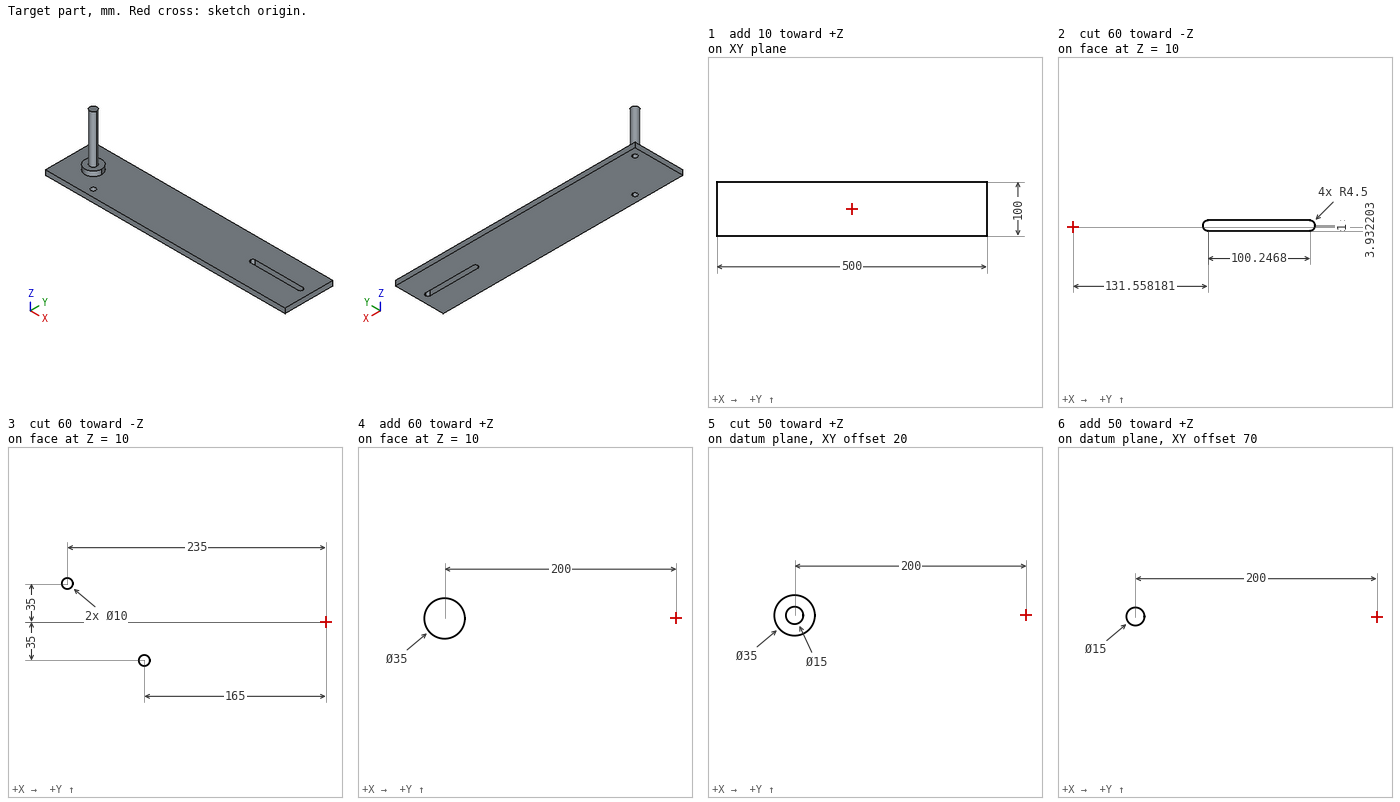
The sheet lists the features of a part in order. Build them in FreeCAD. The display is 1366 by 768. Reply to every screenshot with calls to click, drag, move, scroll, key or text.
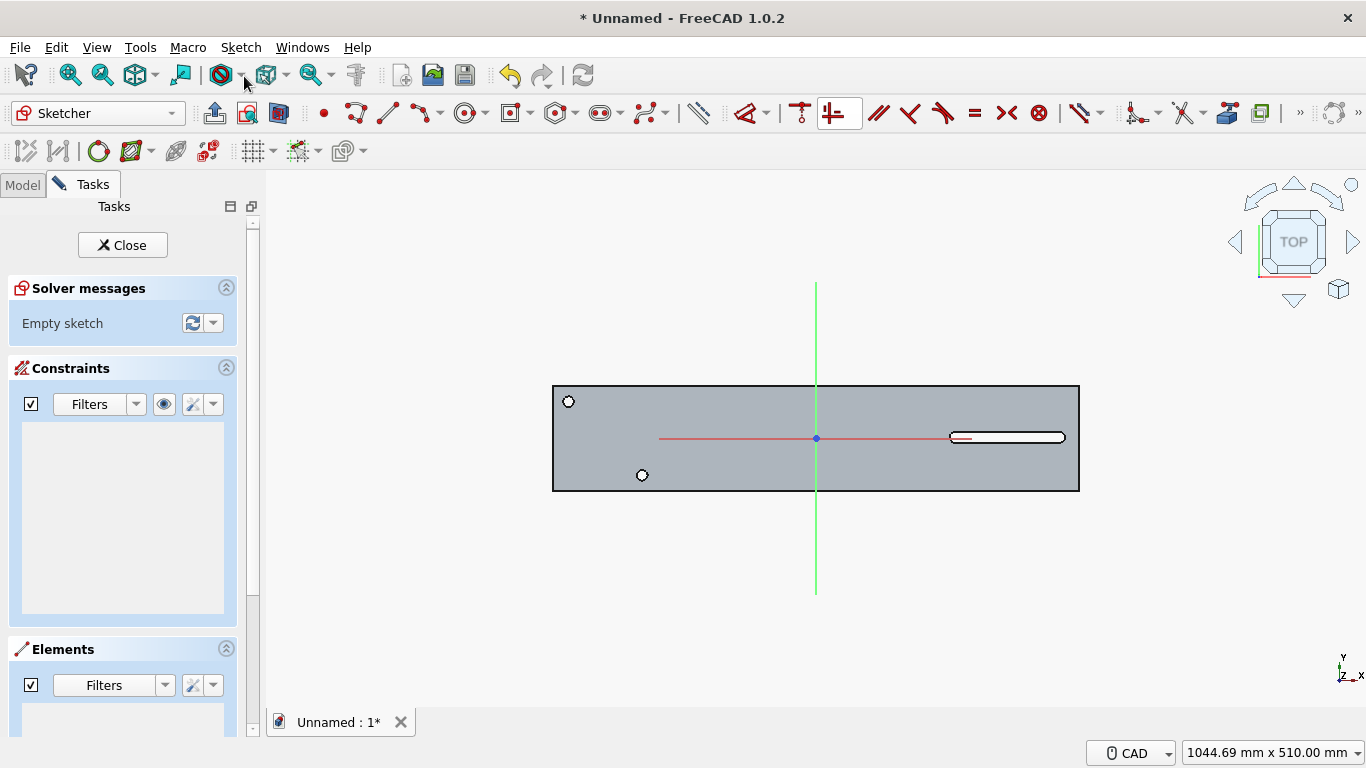
scroll(588, 438, up, 11)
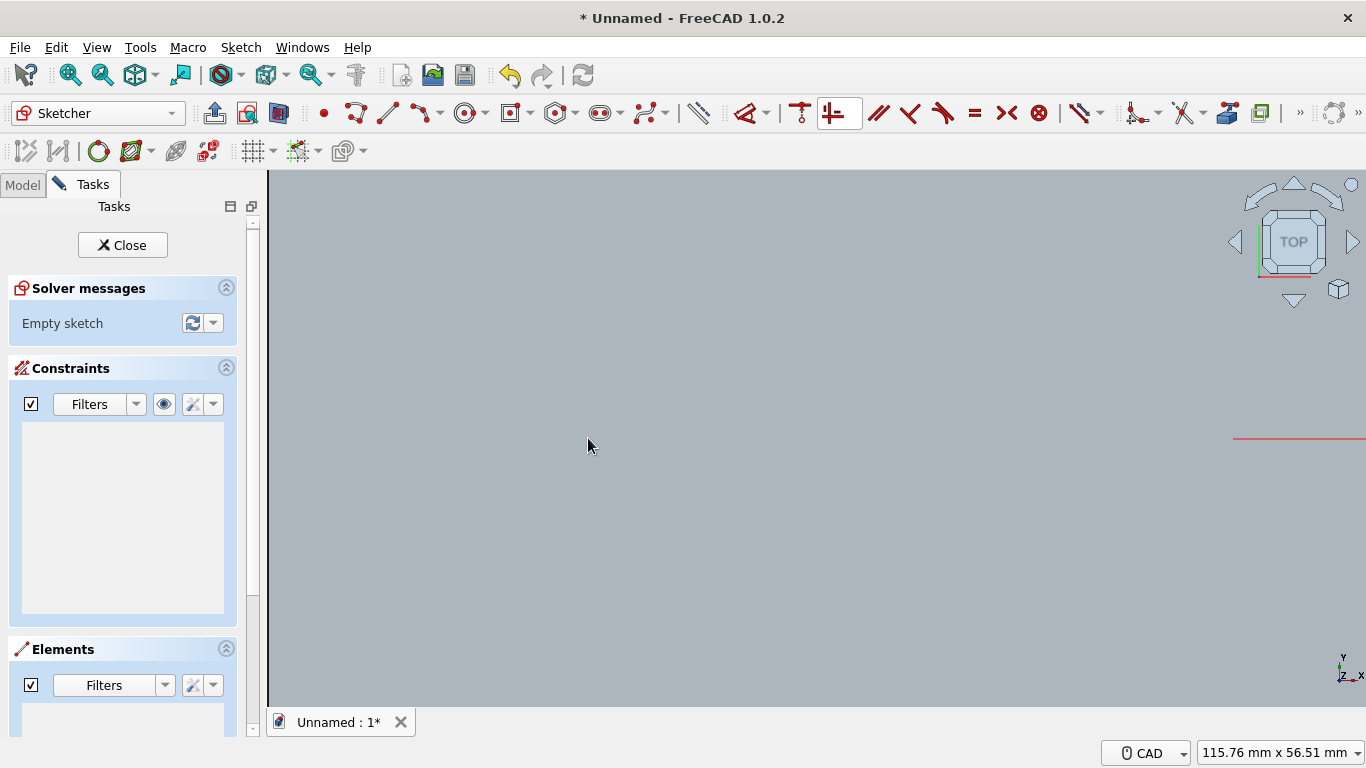
click(466, 114)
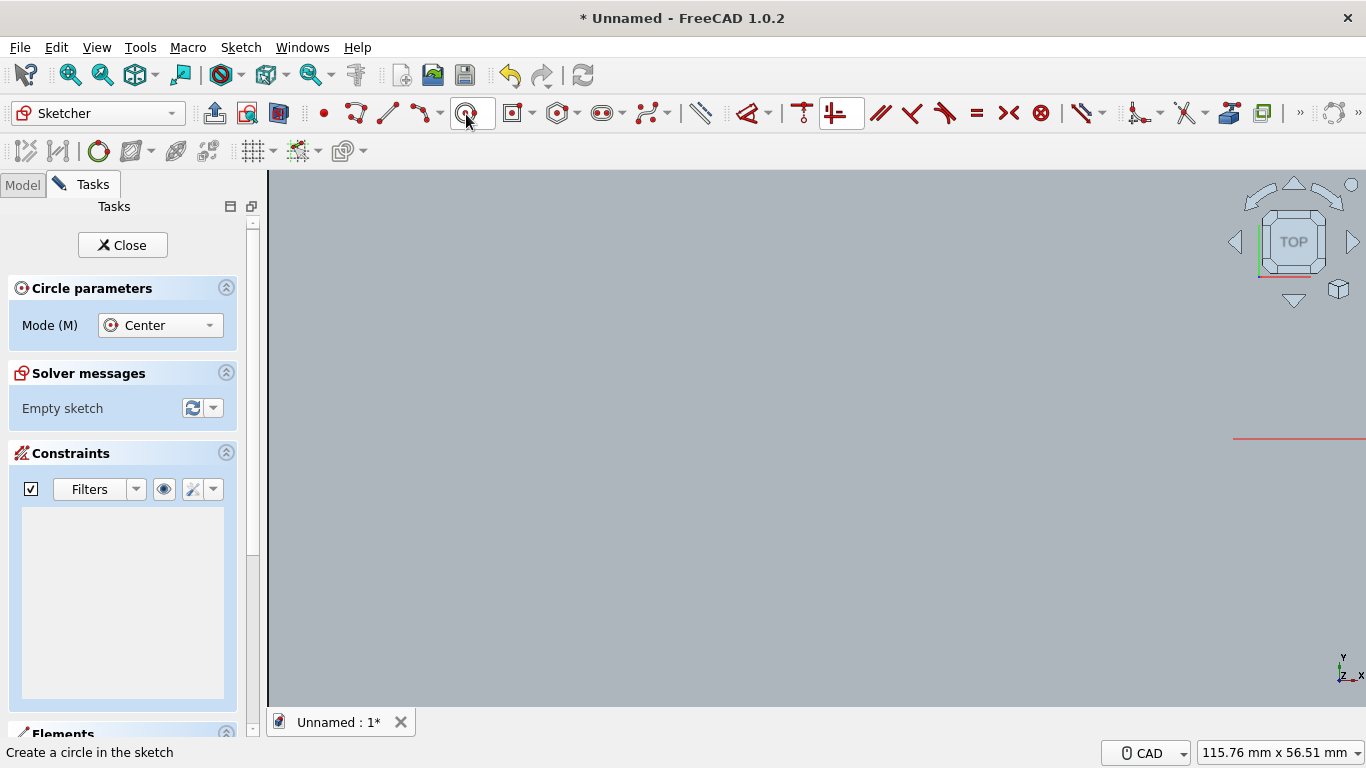
click(743, 438)
move(860, 321)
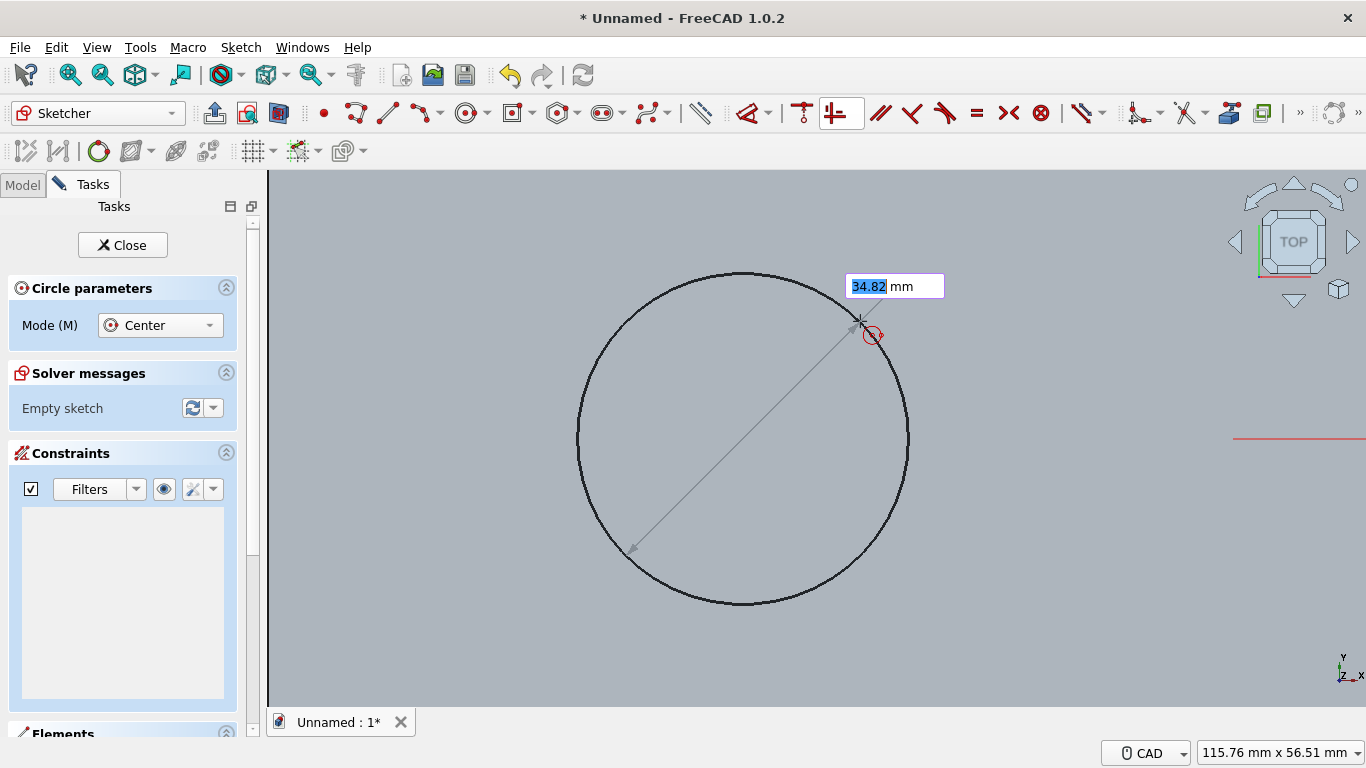
text(35)
key(Return)
key(Escape)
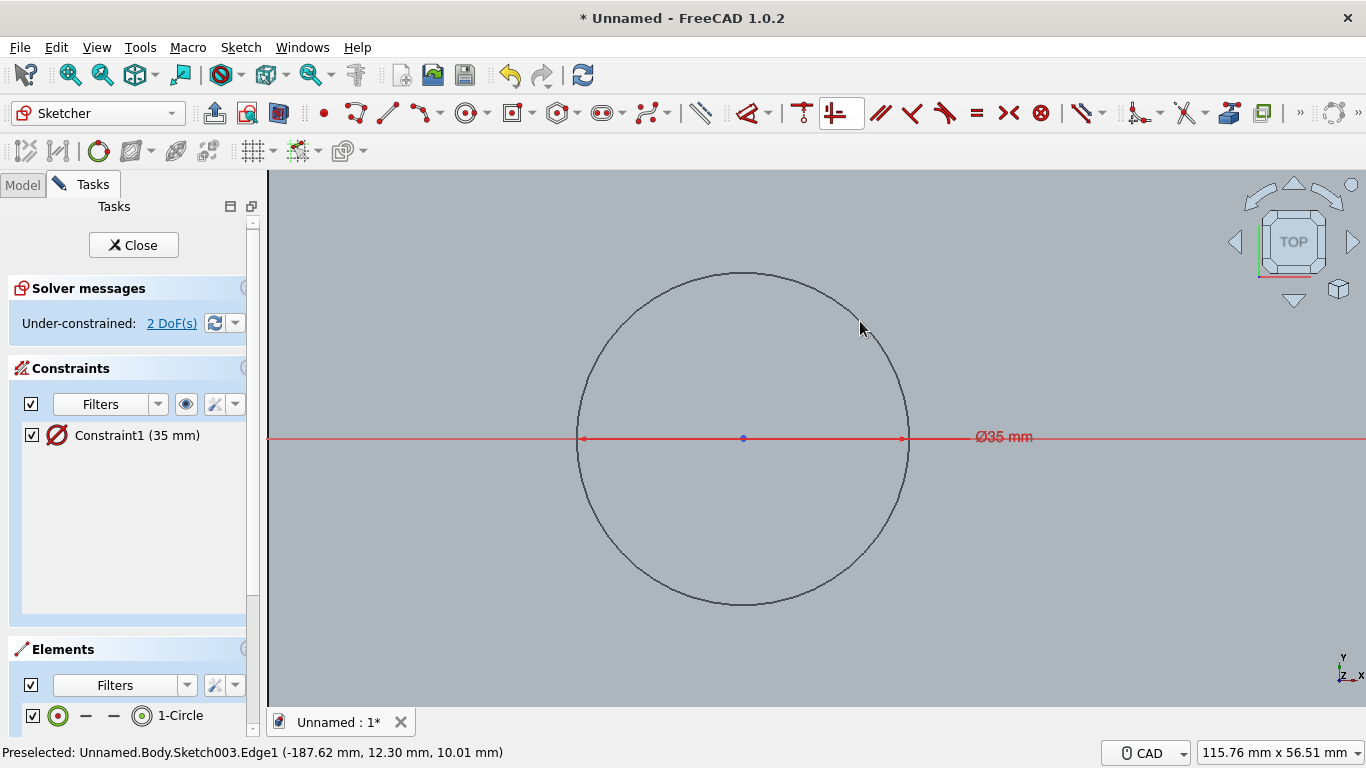
click(743, 439)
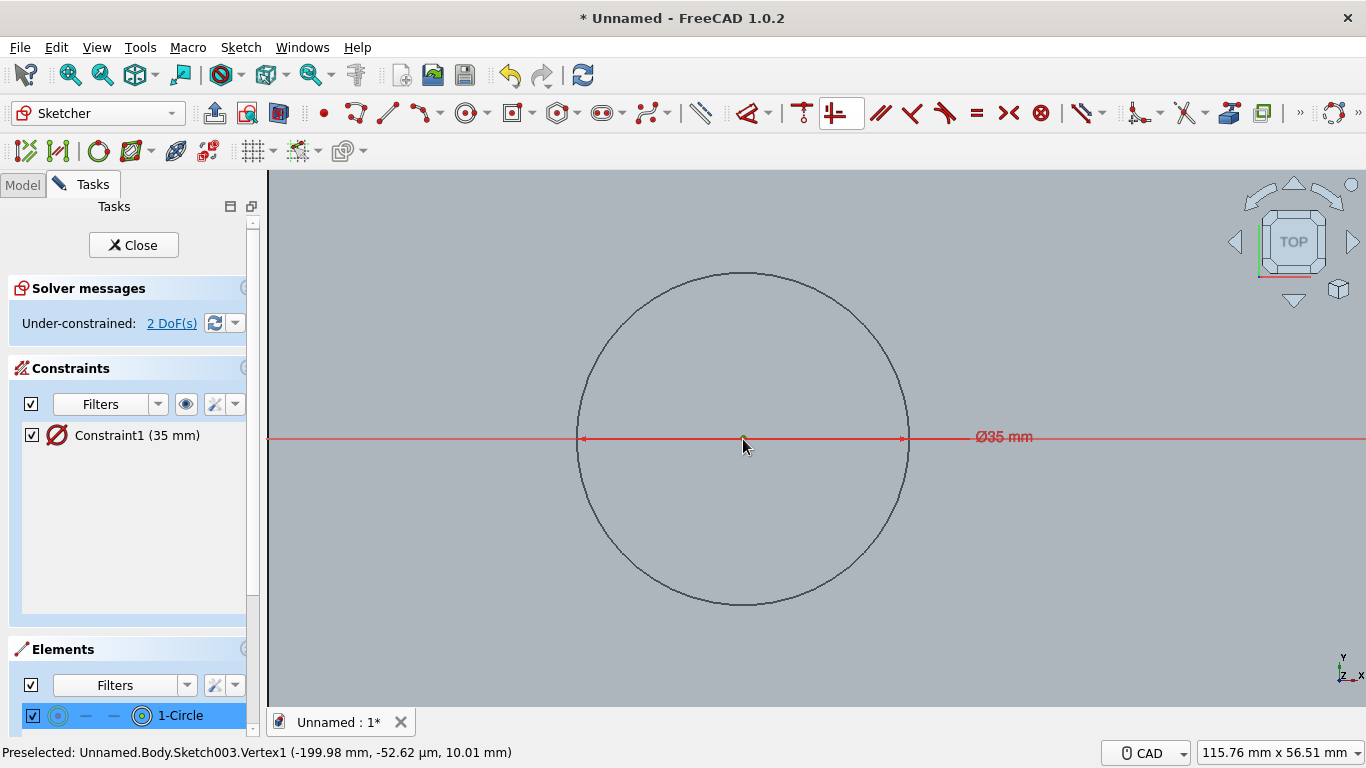
click(359, 438)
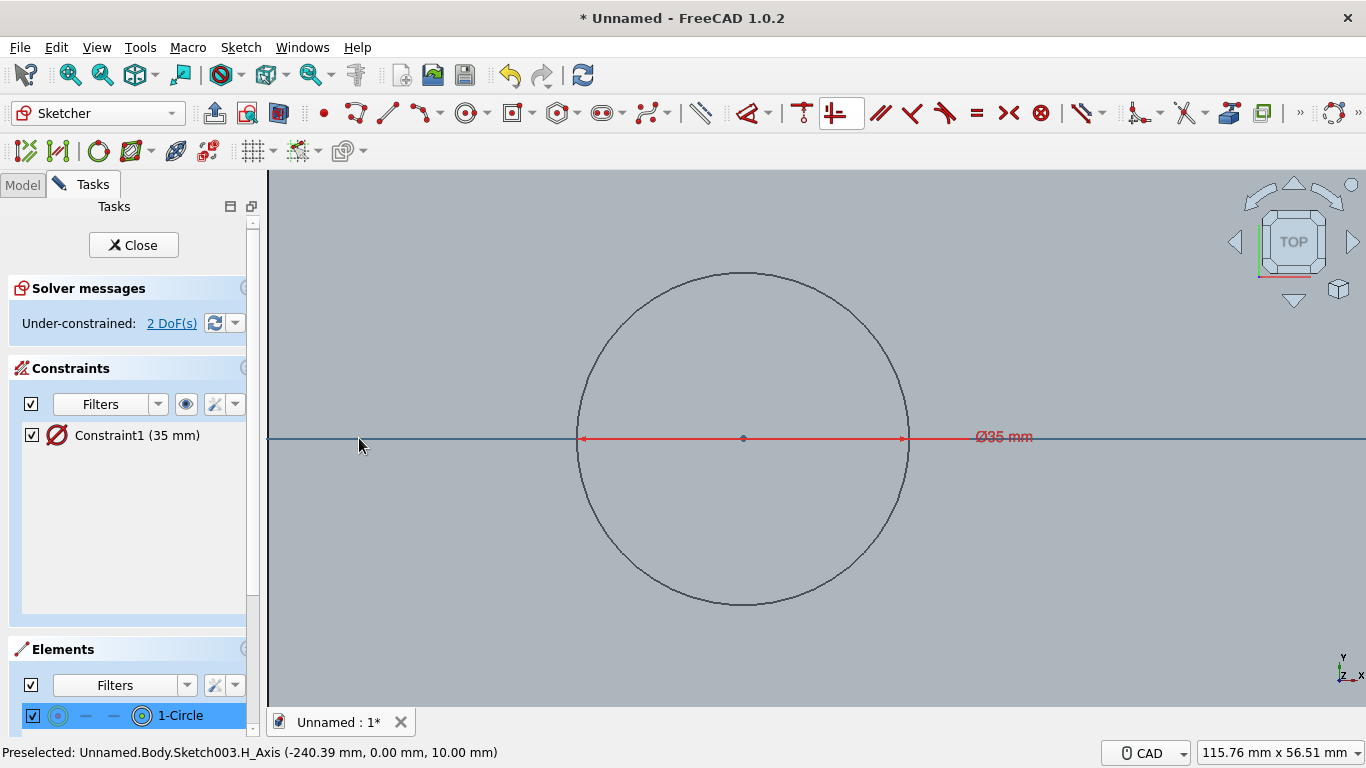
click(802, 114)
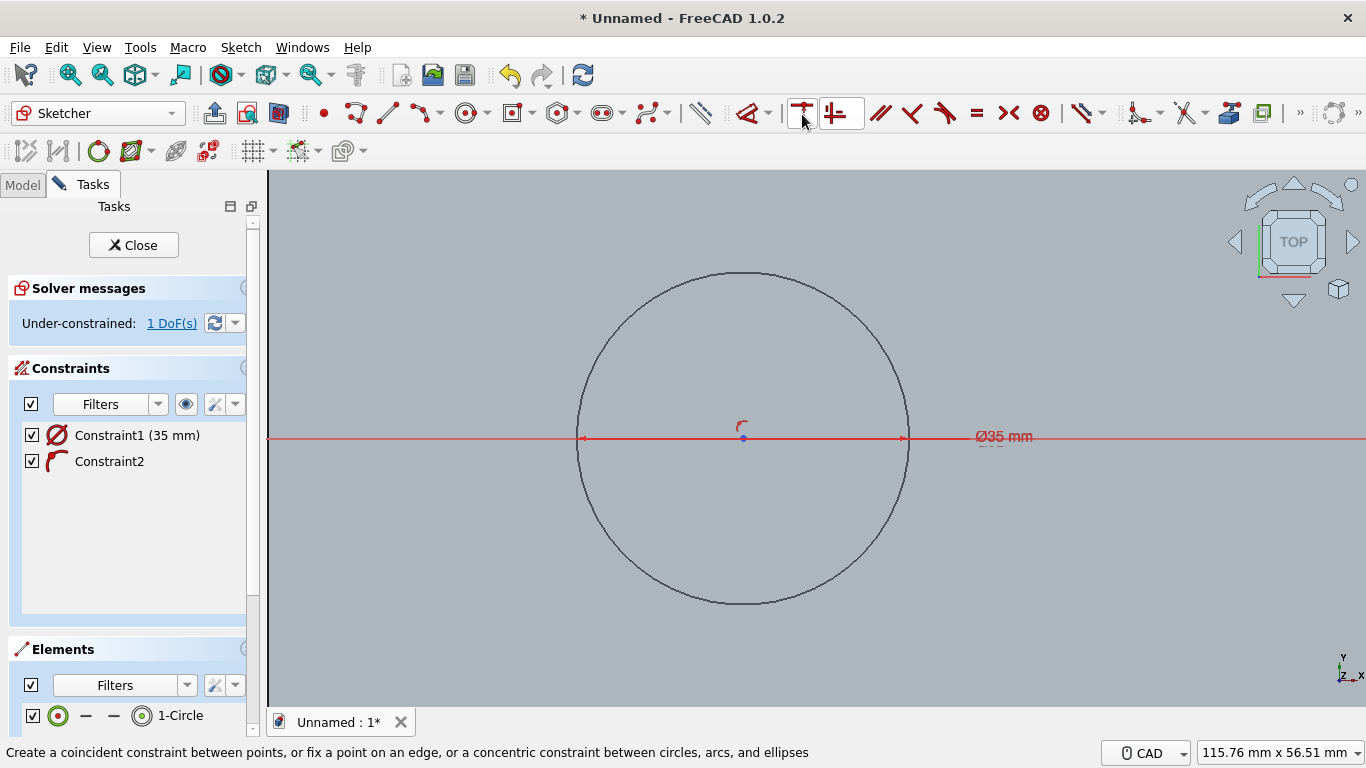
key(d)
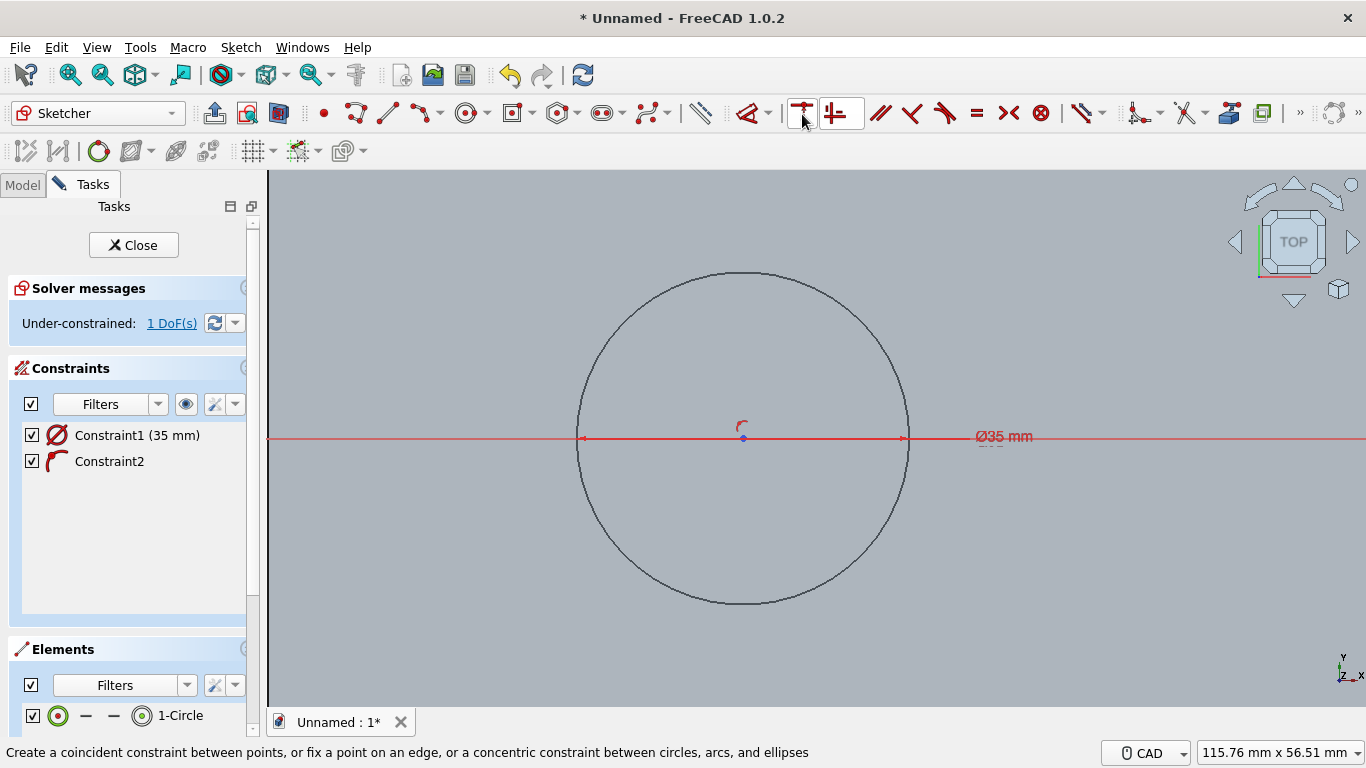
click(743, 438)
click(972, 472)